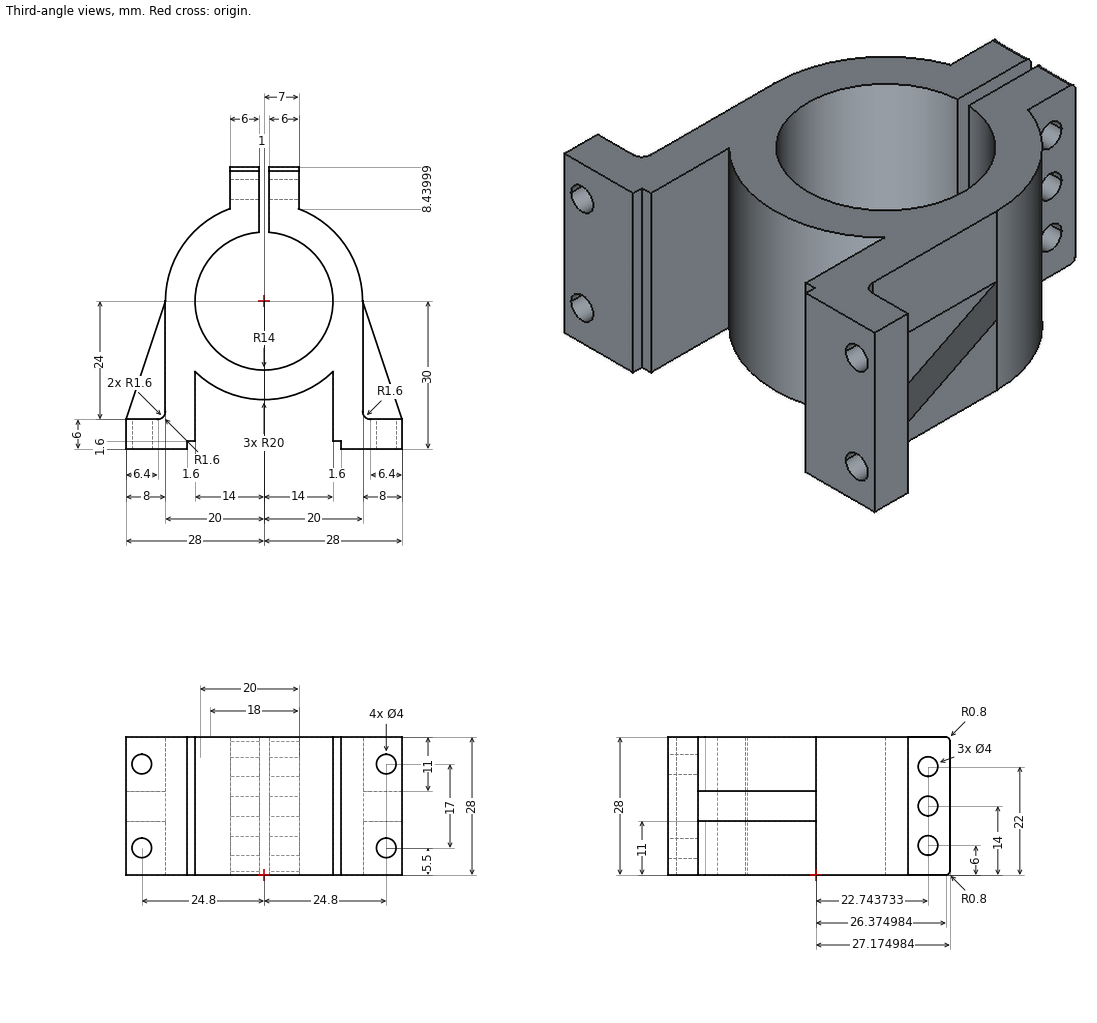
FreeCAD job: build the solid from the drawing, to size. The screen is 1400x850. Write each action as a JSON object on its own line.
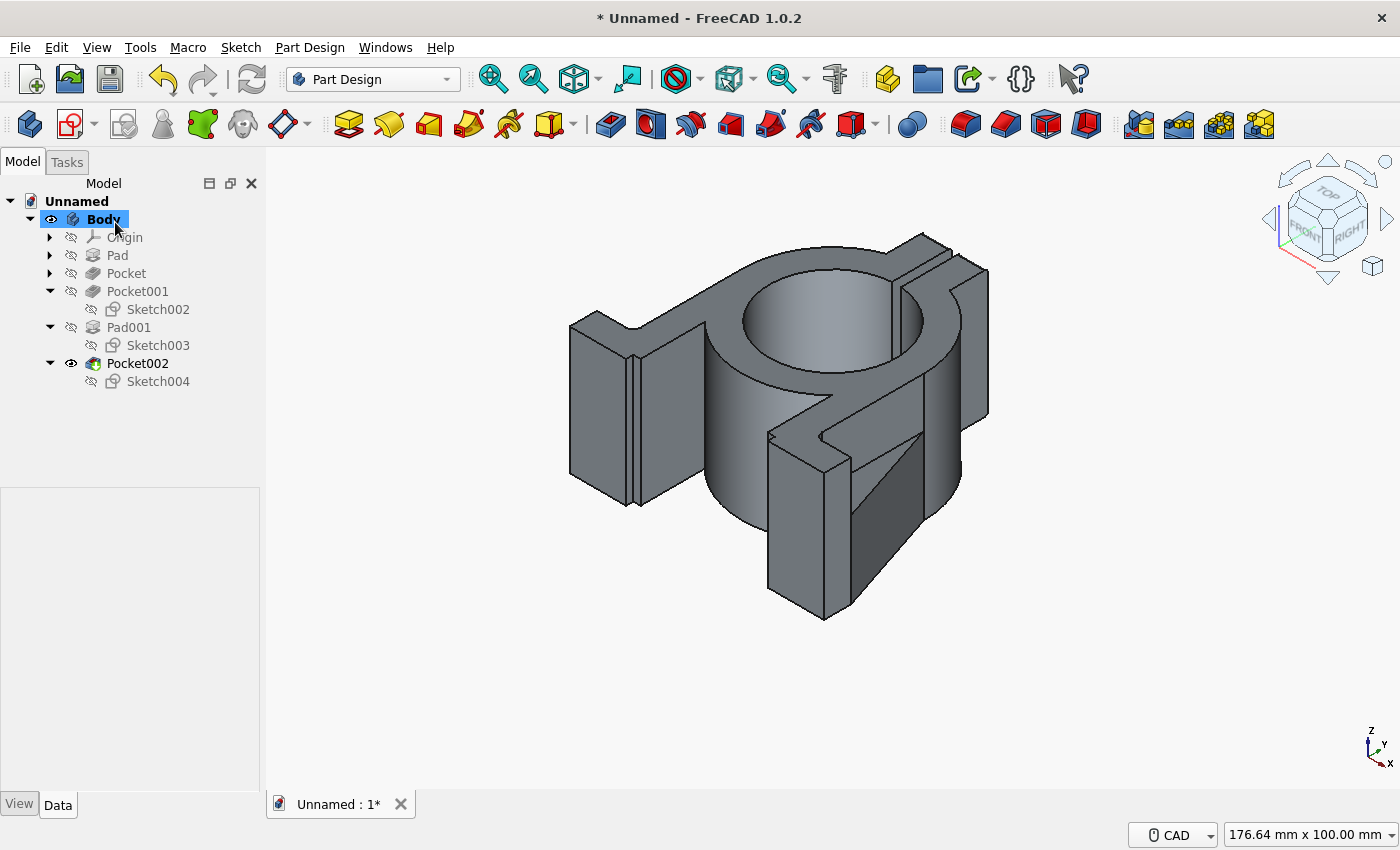
{"action": "left_click", "coordinate": [50, 237]}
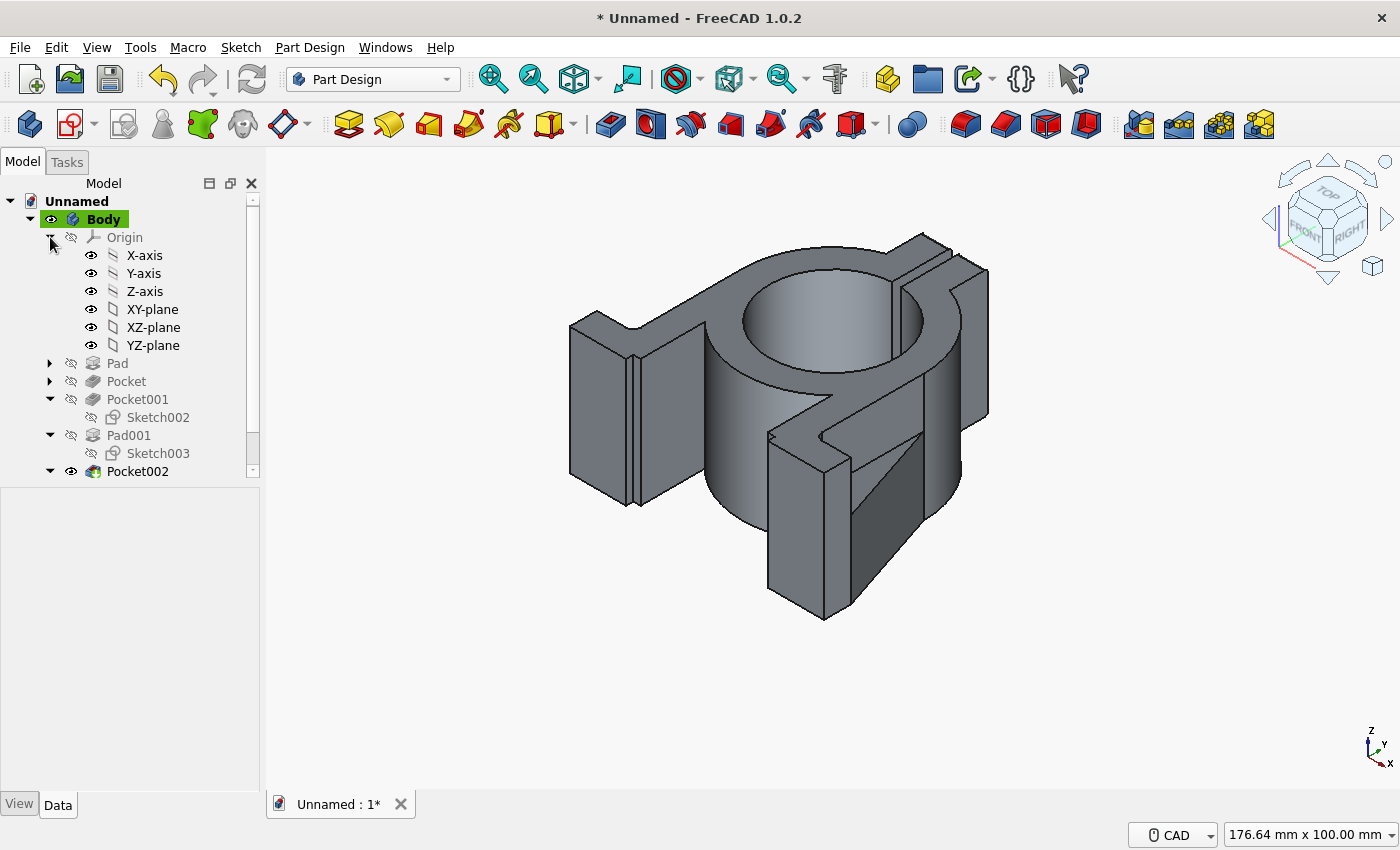
{"action": "left_click", "coordinate": [136, 309]}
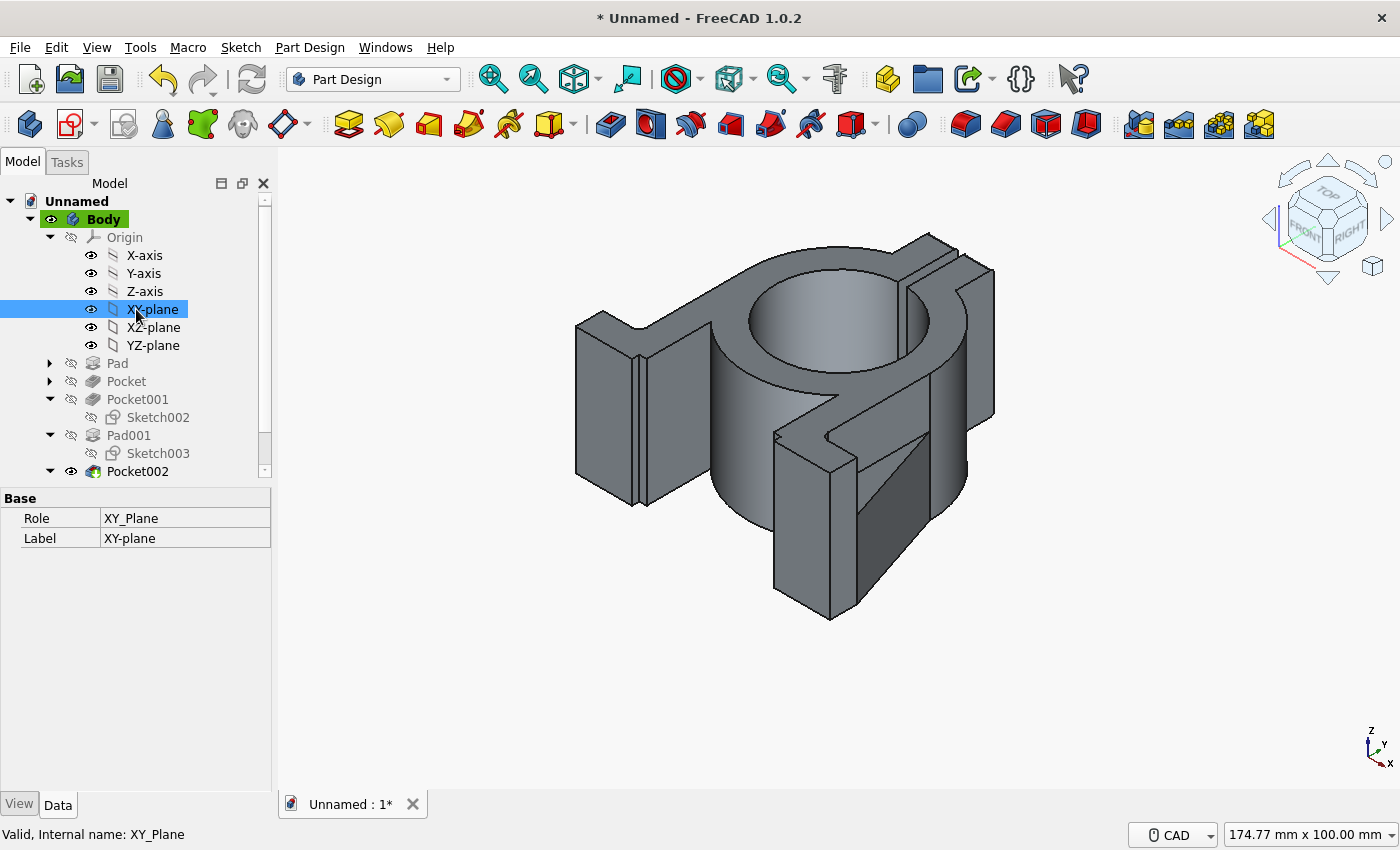
{"action": "left_click", "coordinate": [284, 124]}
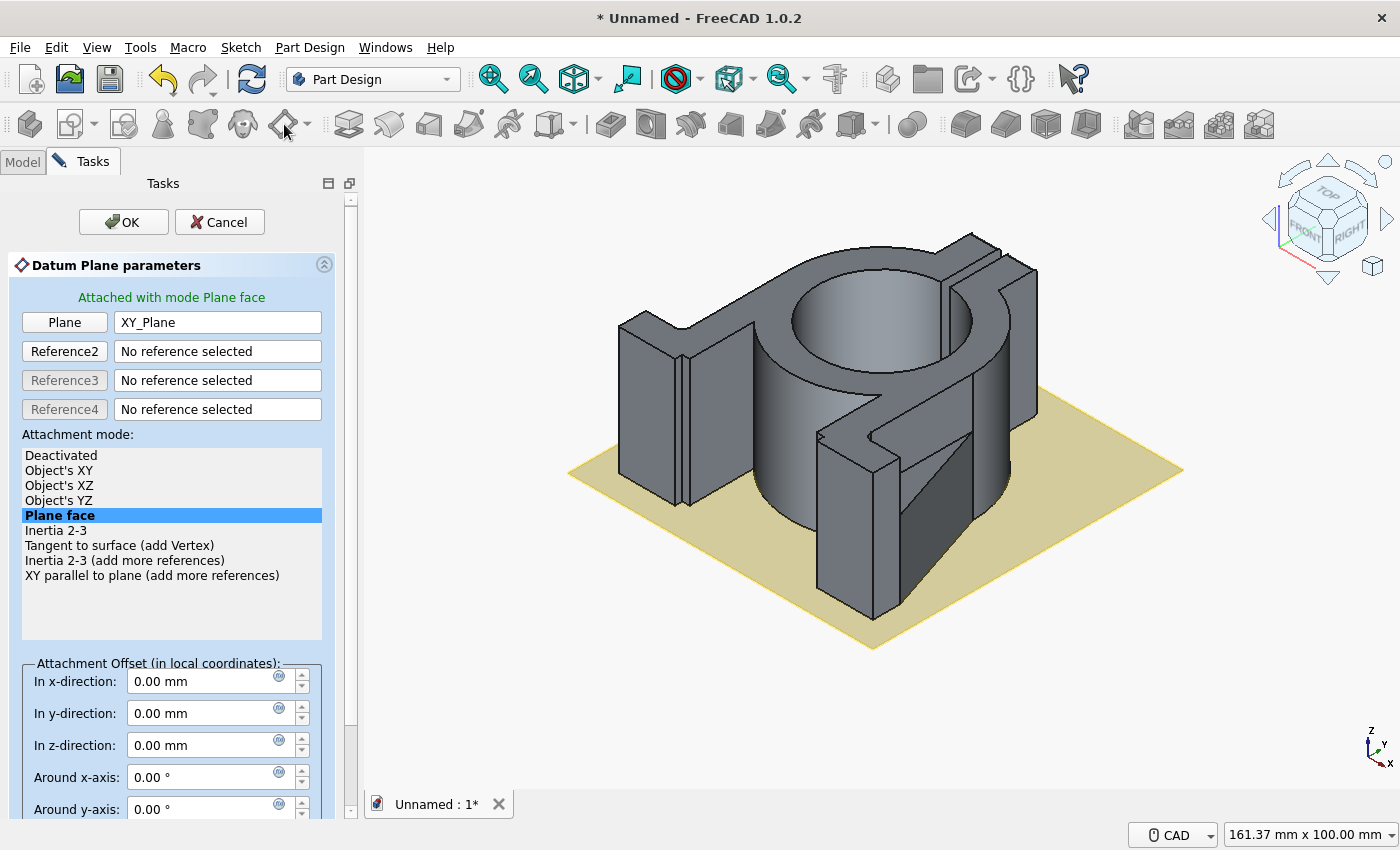
{"action": "triple_click", "coordinate": [210, 745]}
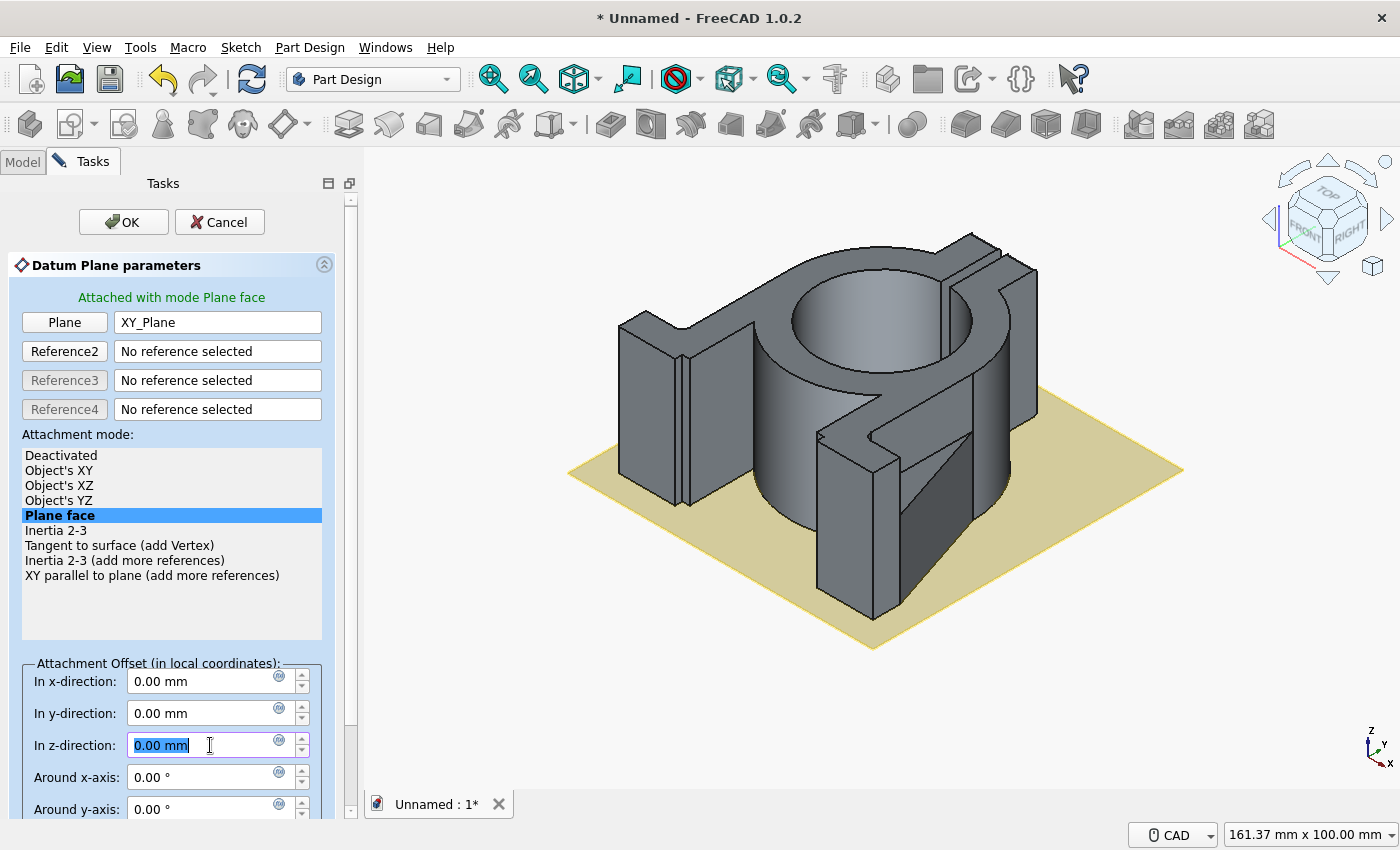
{"action": "type", "text": "11"}
{"action": "key", "text": "Tab"}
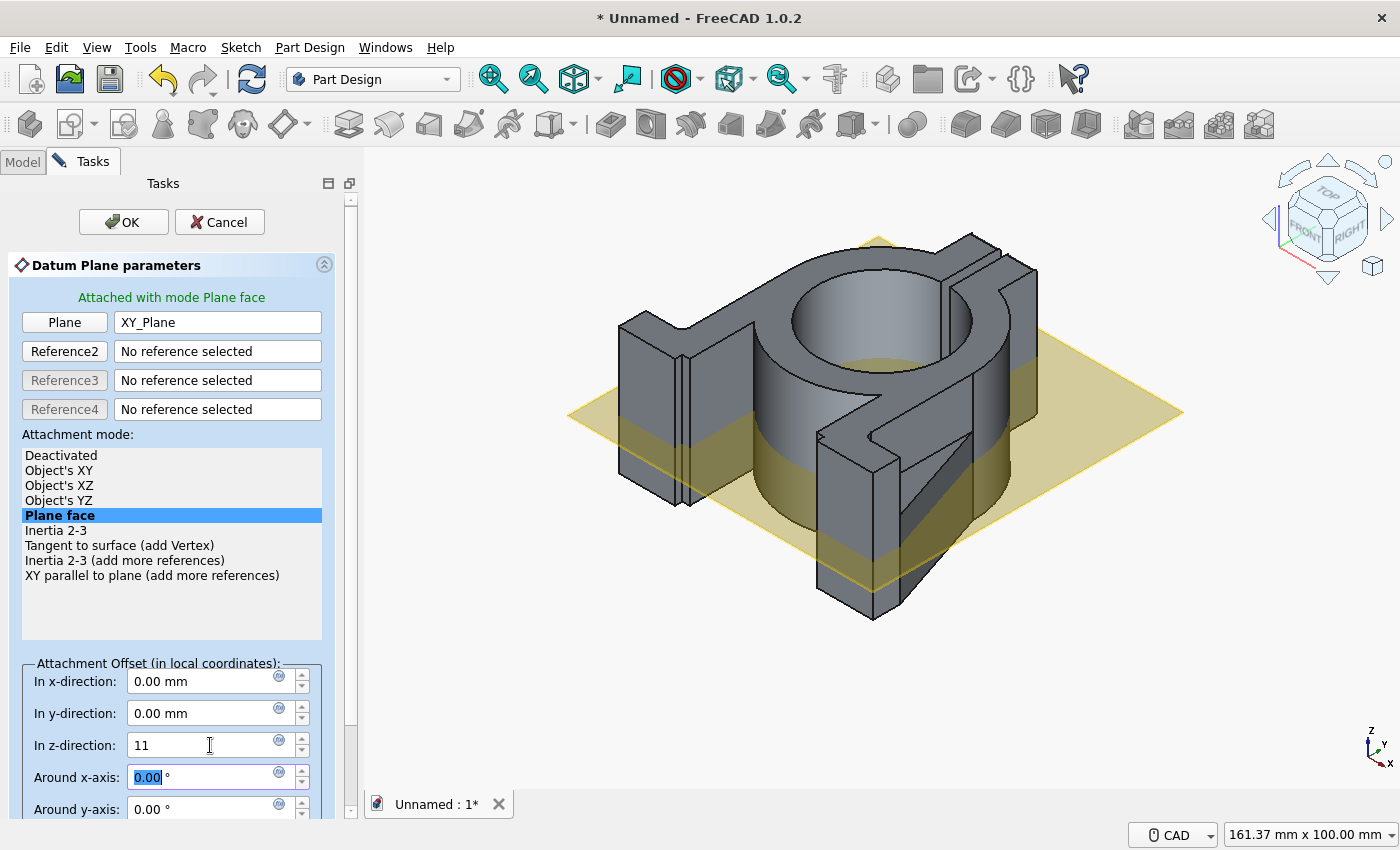
{"action": "left_click", "coordinate": [124, 222]}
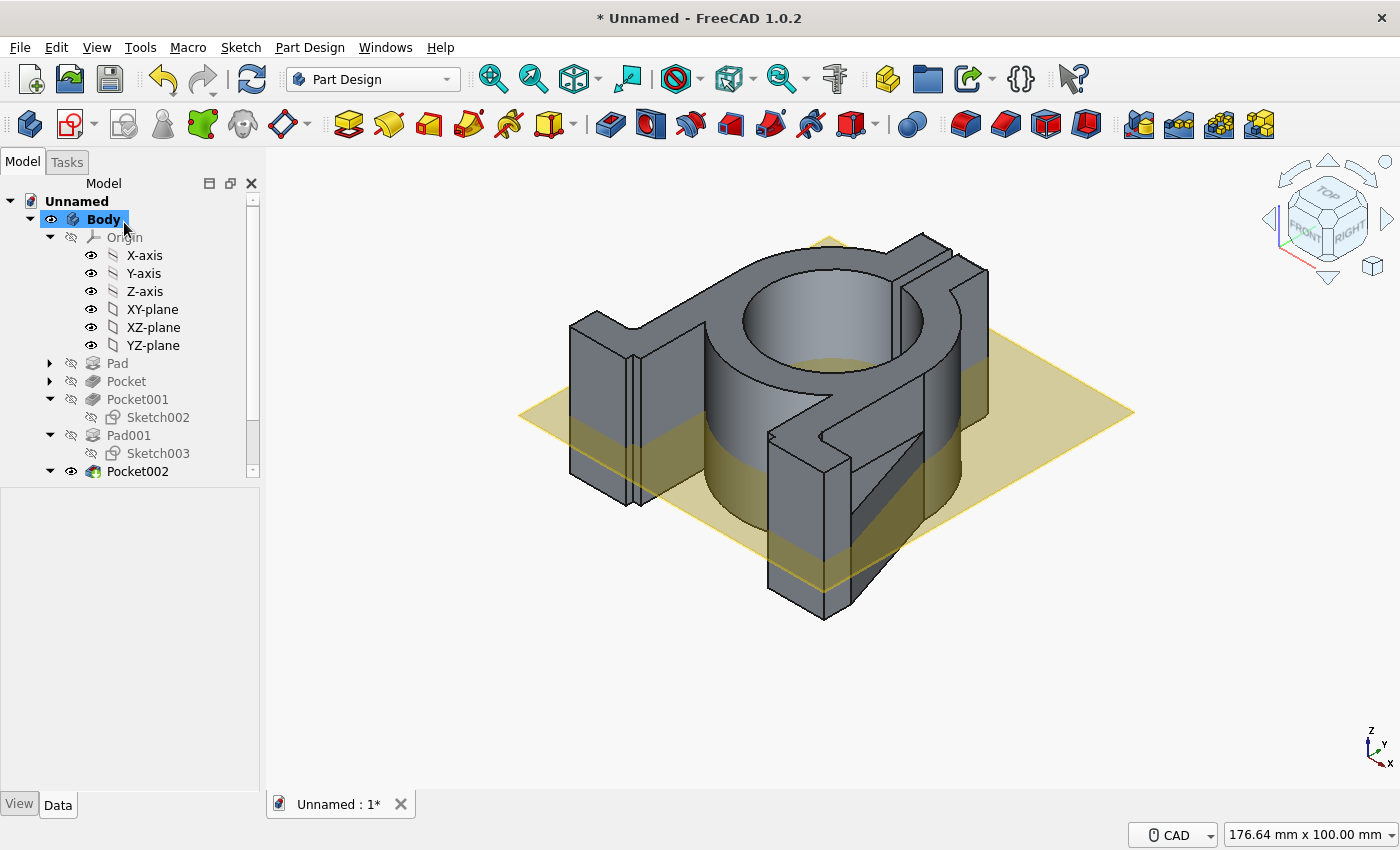
{"action": "scroll", "coordinate": [100, 341], "scroll_direction": "down", "scroll_amount": 3}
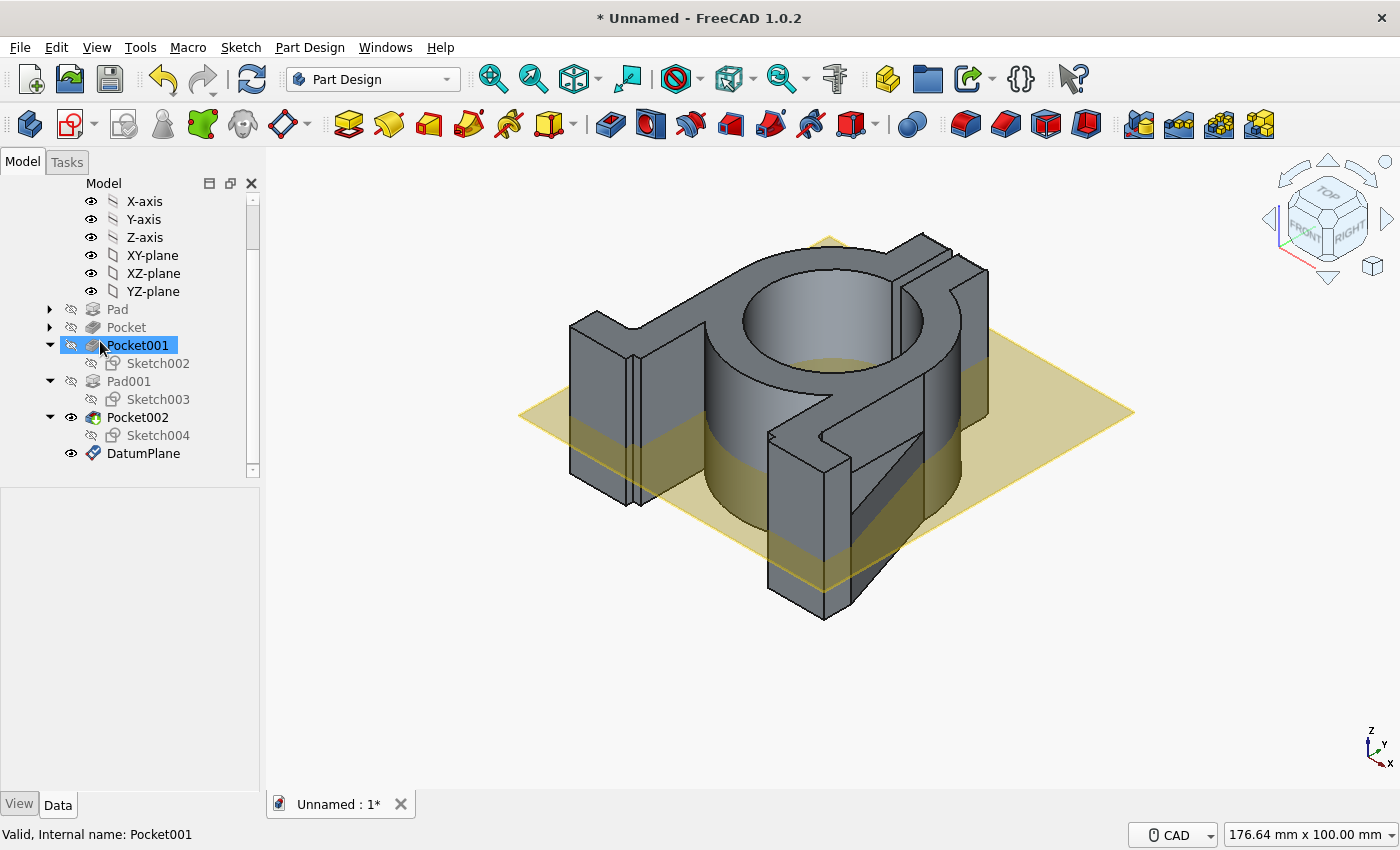
{"action": "left_click", "coordinate": [116, 453]}